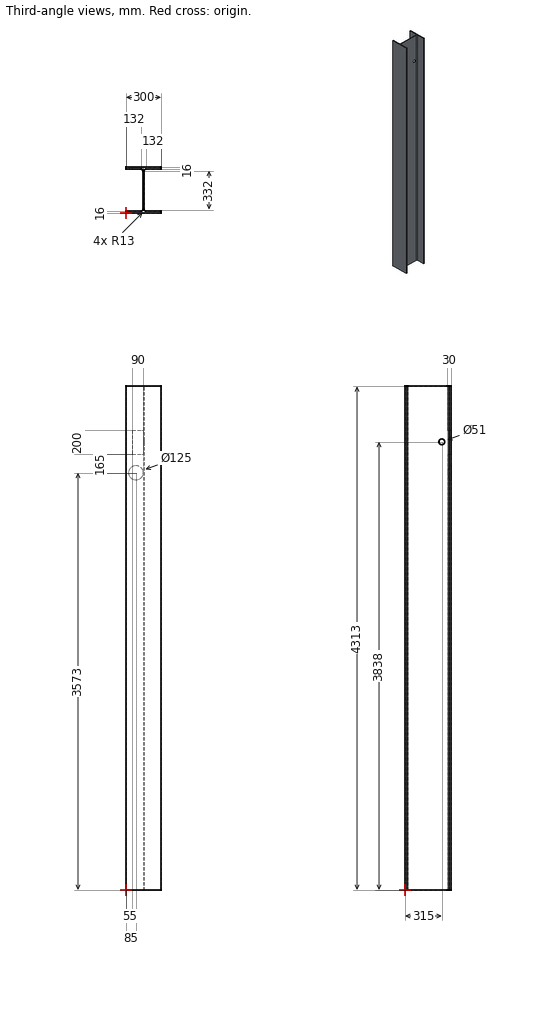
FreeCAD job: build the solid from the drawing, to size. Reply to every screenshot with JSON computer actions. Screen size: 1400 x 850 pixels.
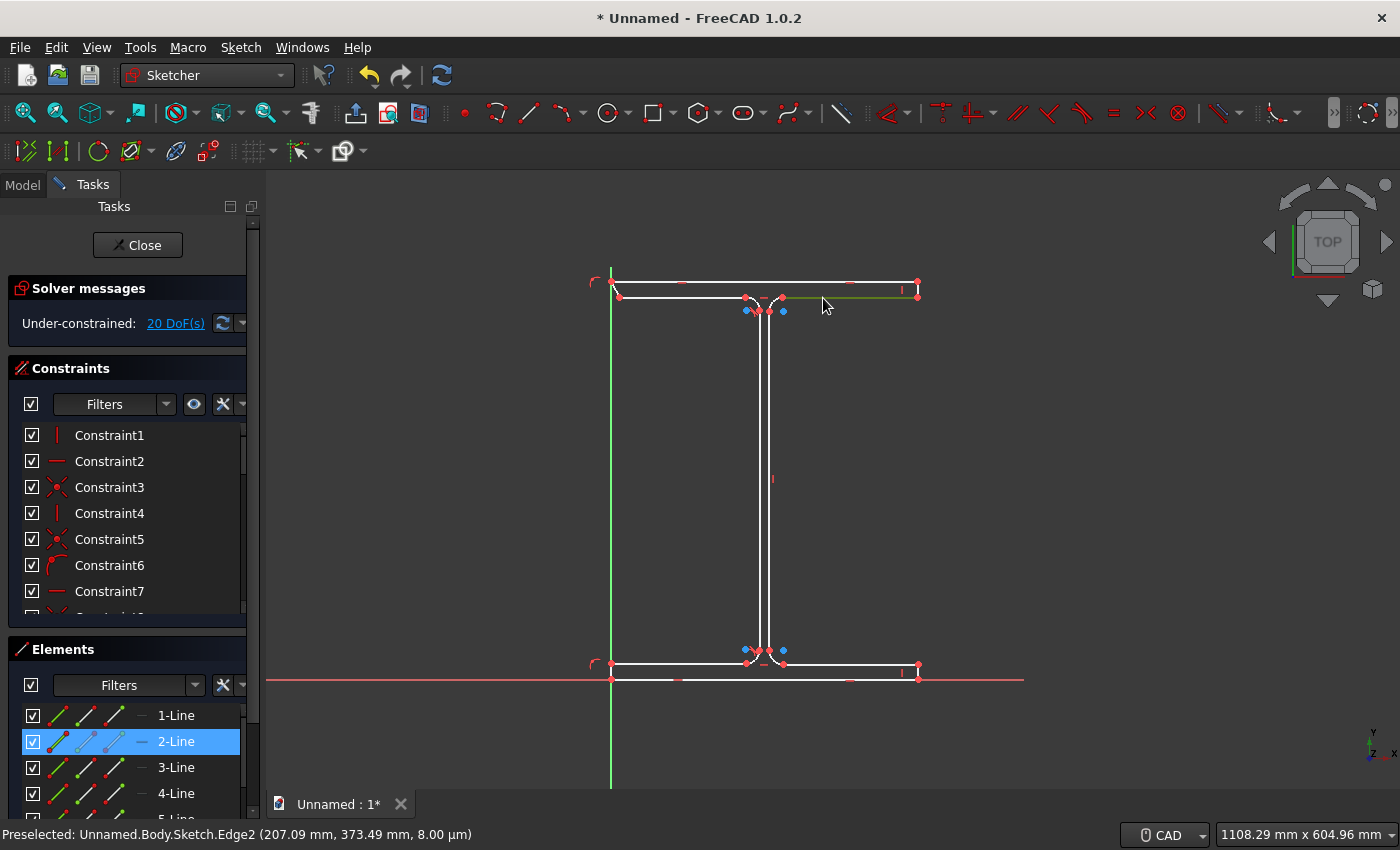
{"action": "scroll", "coordinate": [773, 302], "scroll_direction": "up", "scroll_amount": 2}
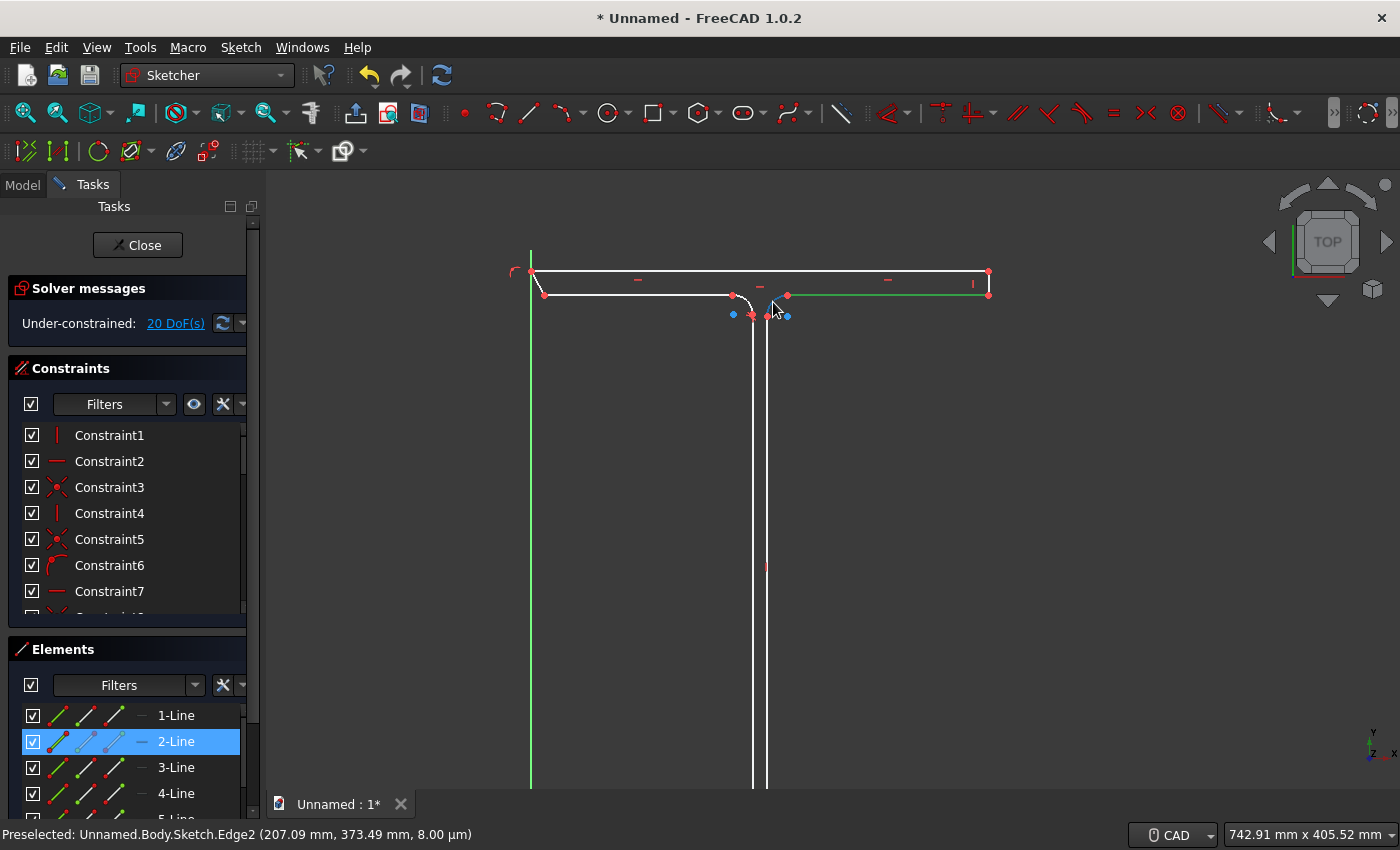
{"action": "left_click", "coordinate": [773, 302]}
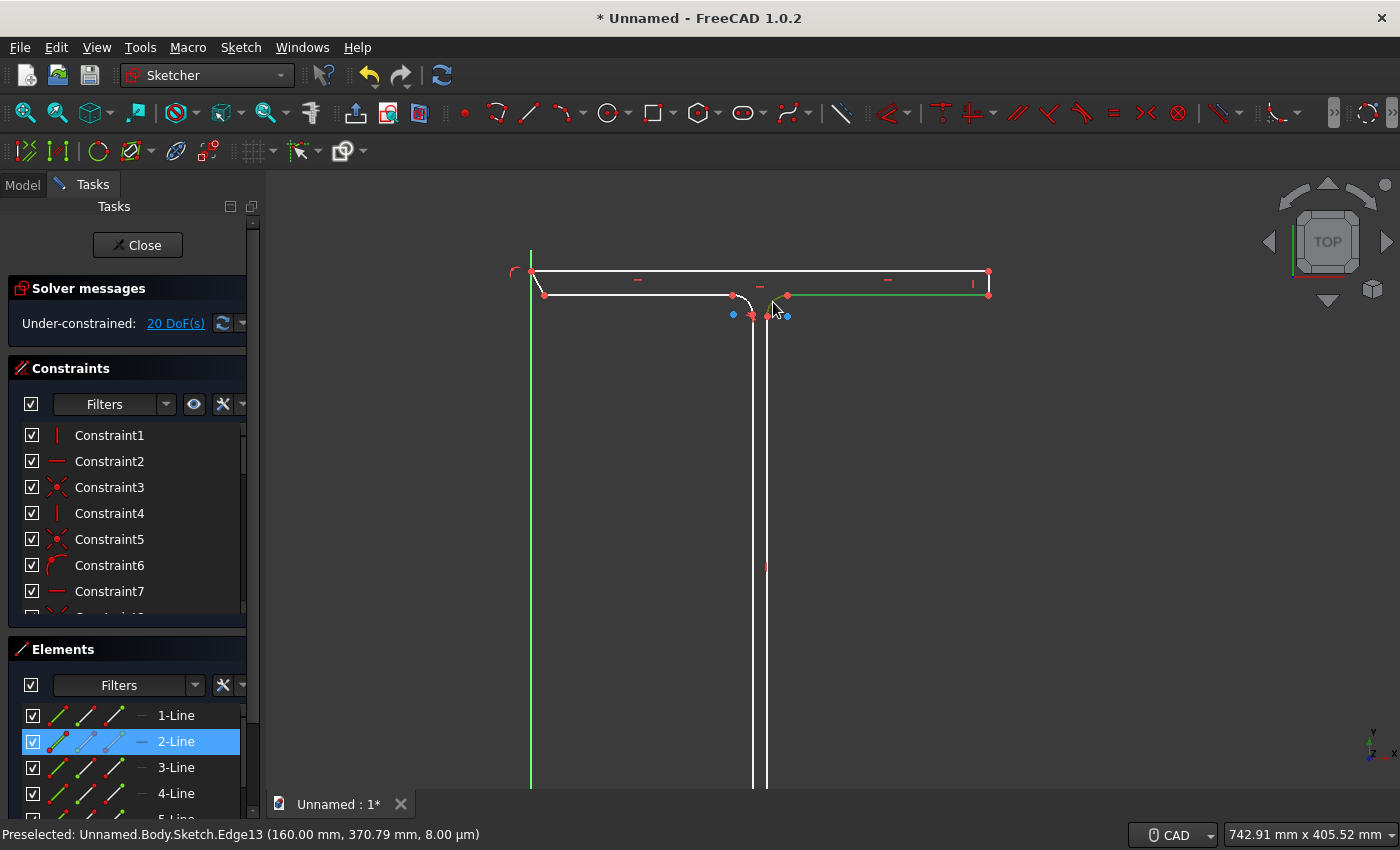
{"action": "left_click", "coordinate": [1082, 114]}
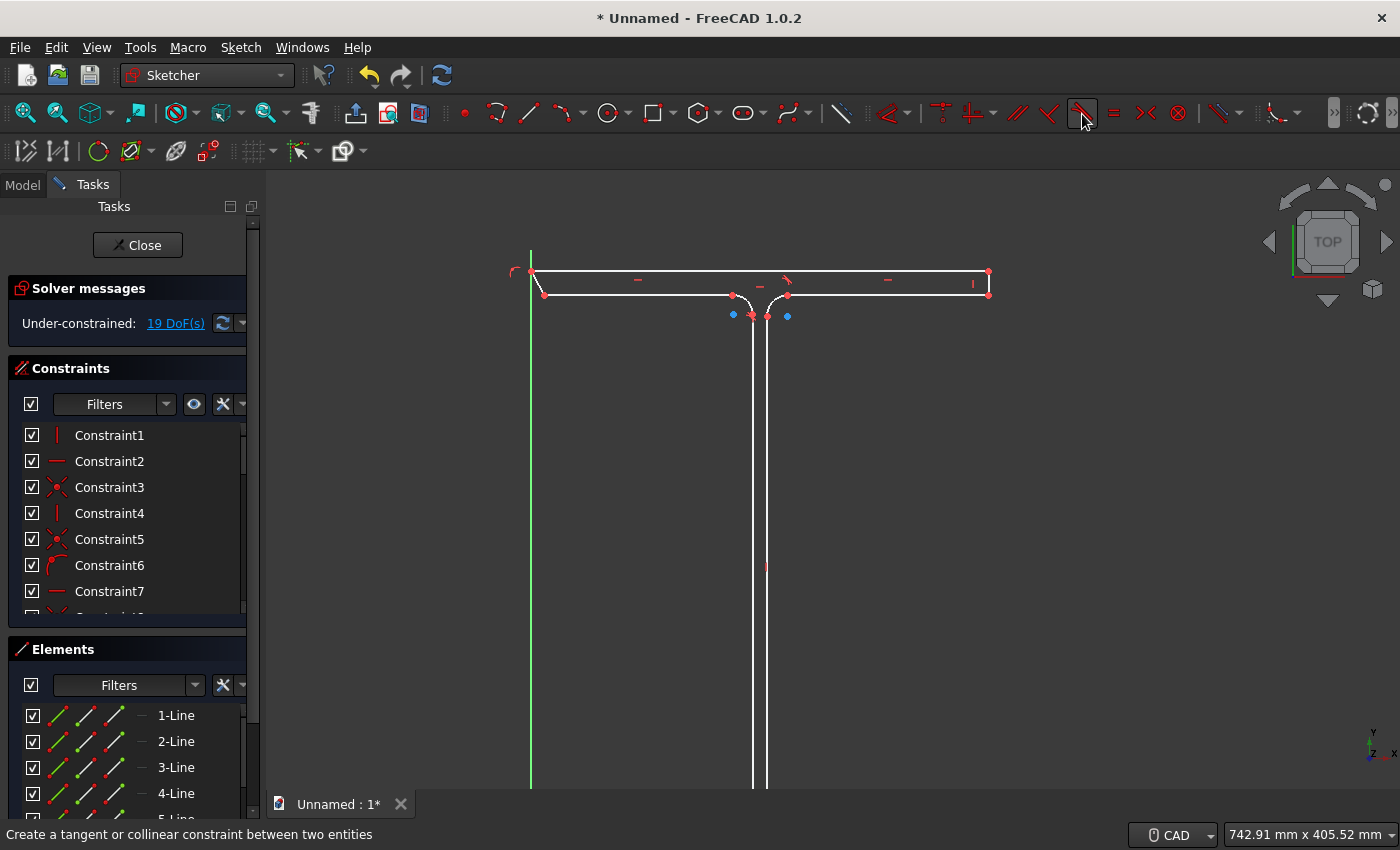
{"action": "left_click", "coordinate": [601, 295]}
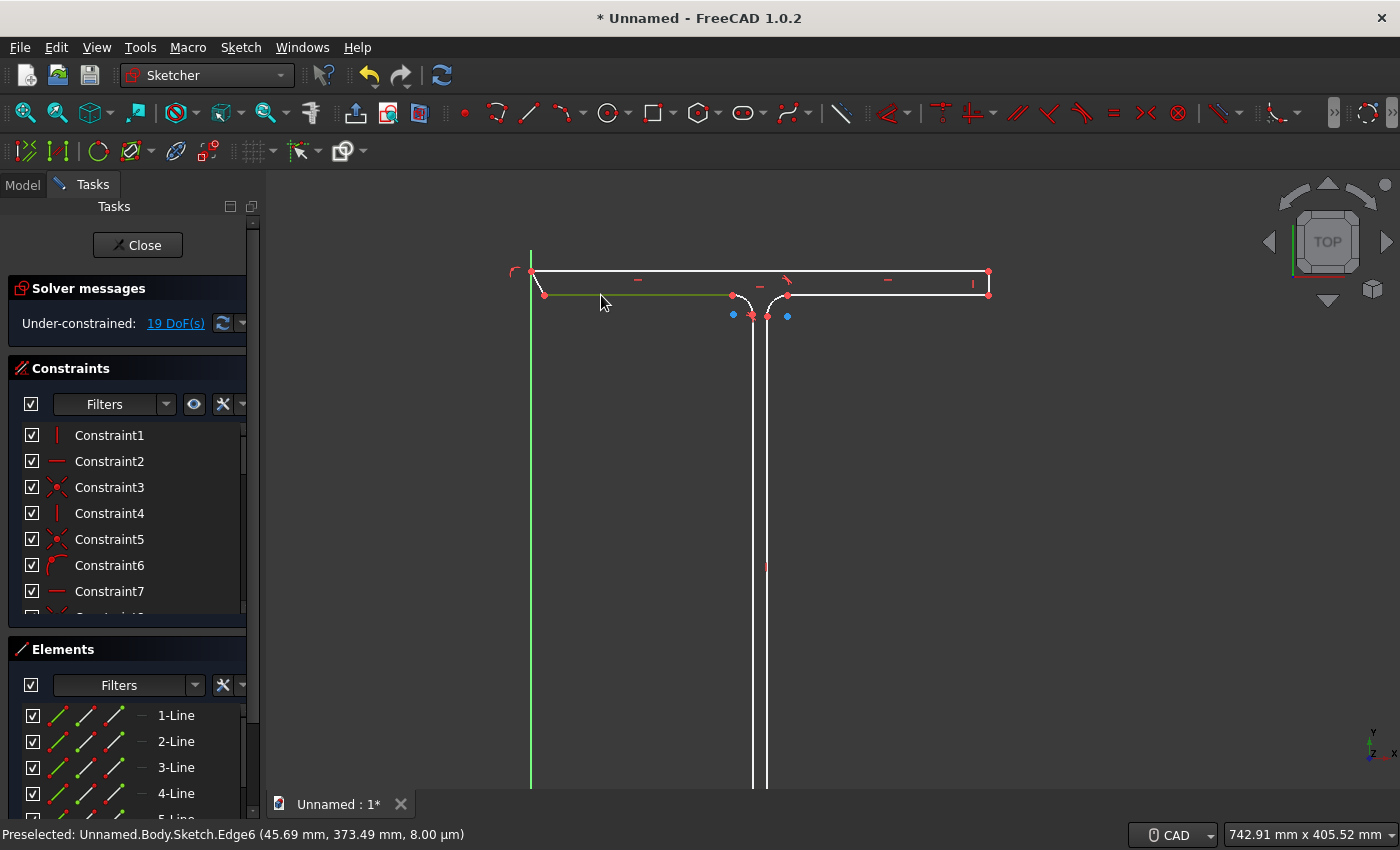
{"action": "scroll", "coordinate": [751, 306], "scroll_direction": "up", "scroll_amount": 2}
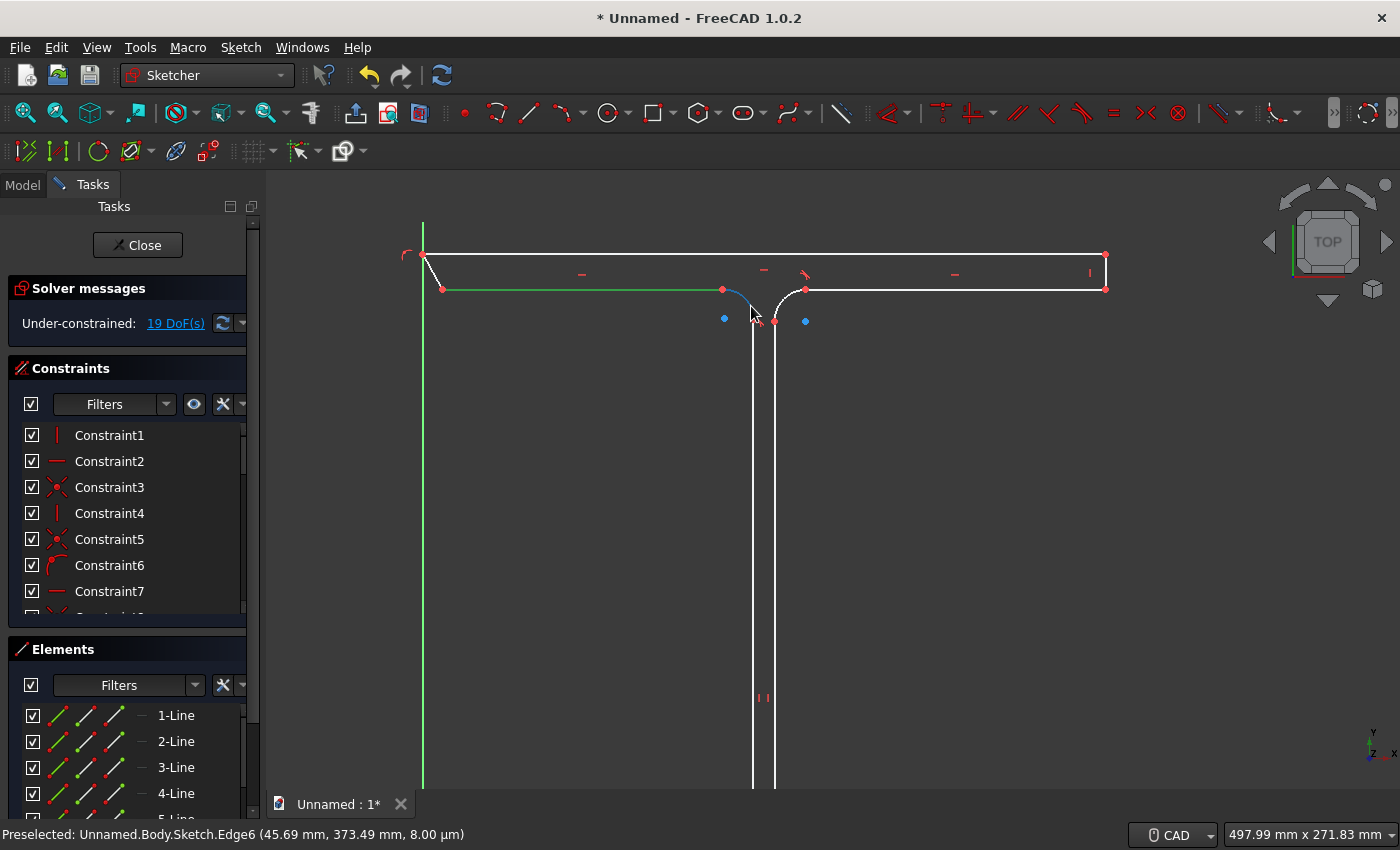
{"action": "left_click", "coordinate": [750, 305]}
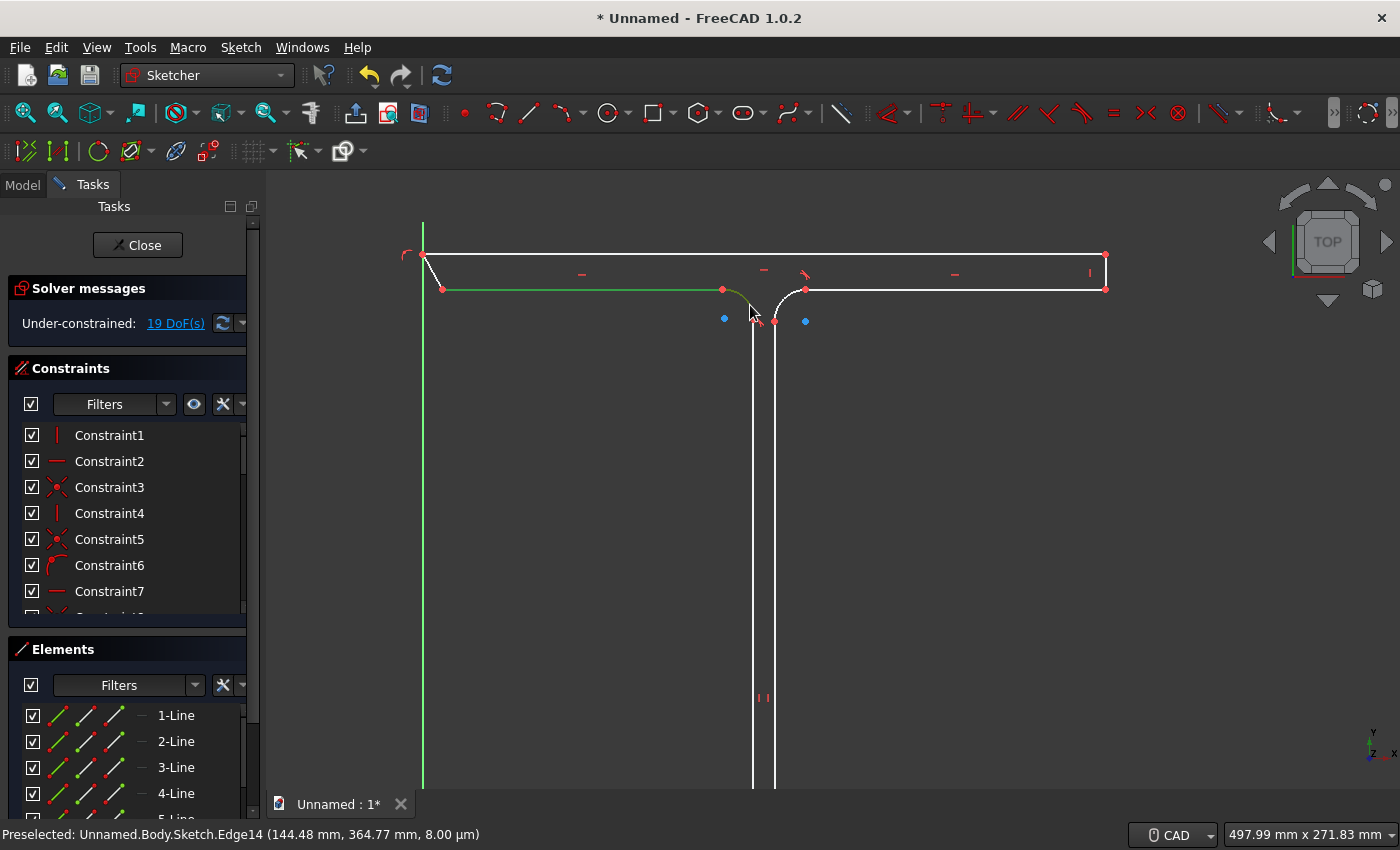
{"action": "left_click", "coordinate": [1082, 114]}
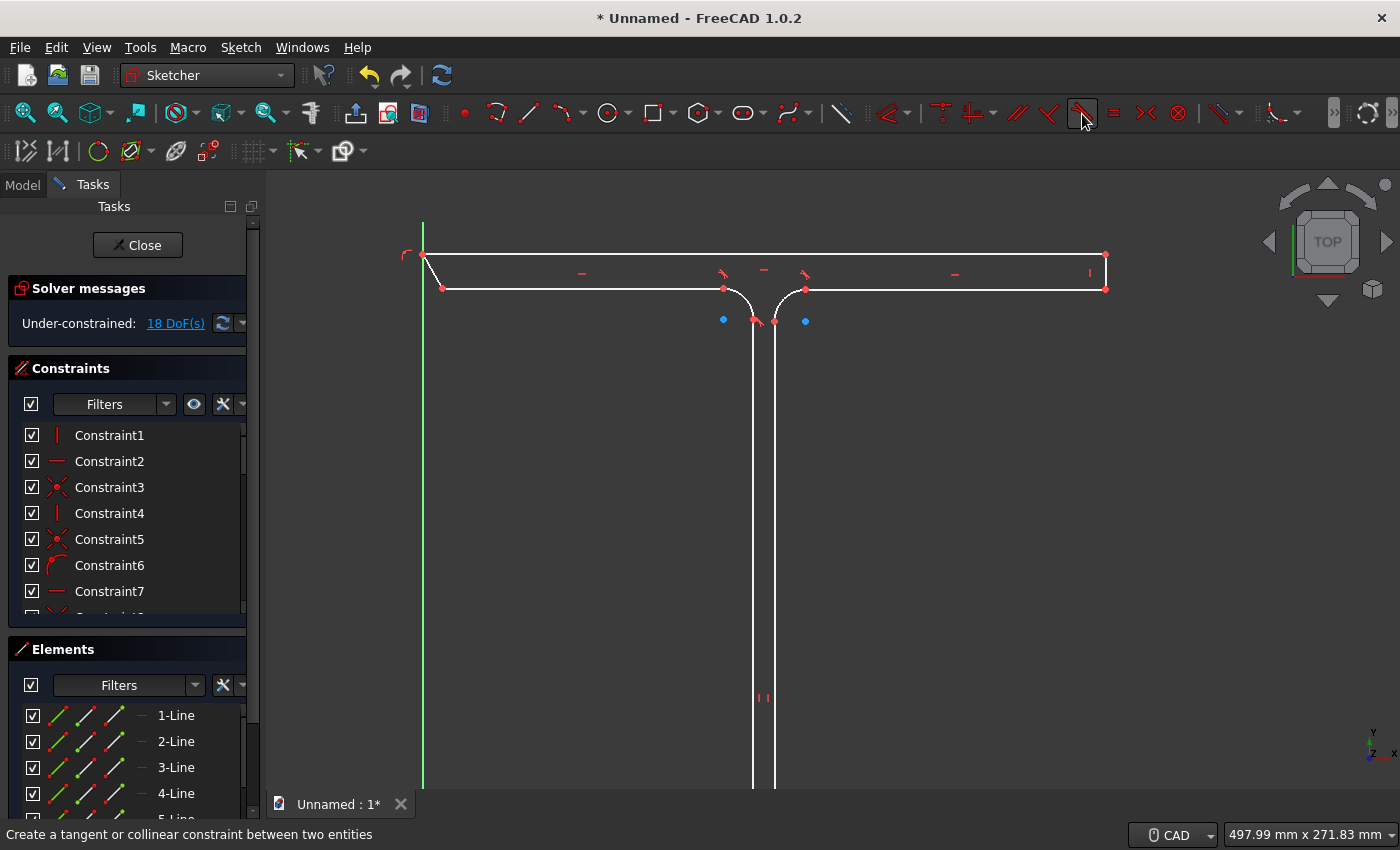
{"action": "left_click", "coordinate": [753, 546]}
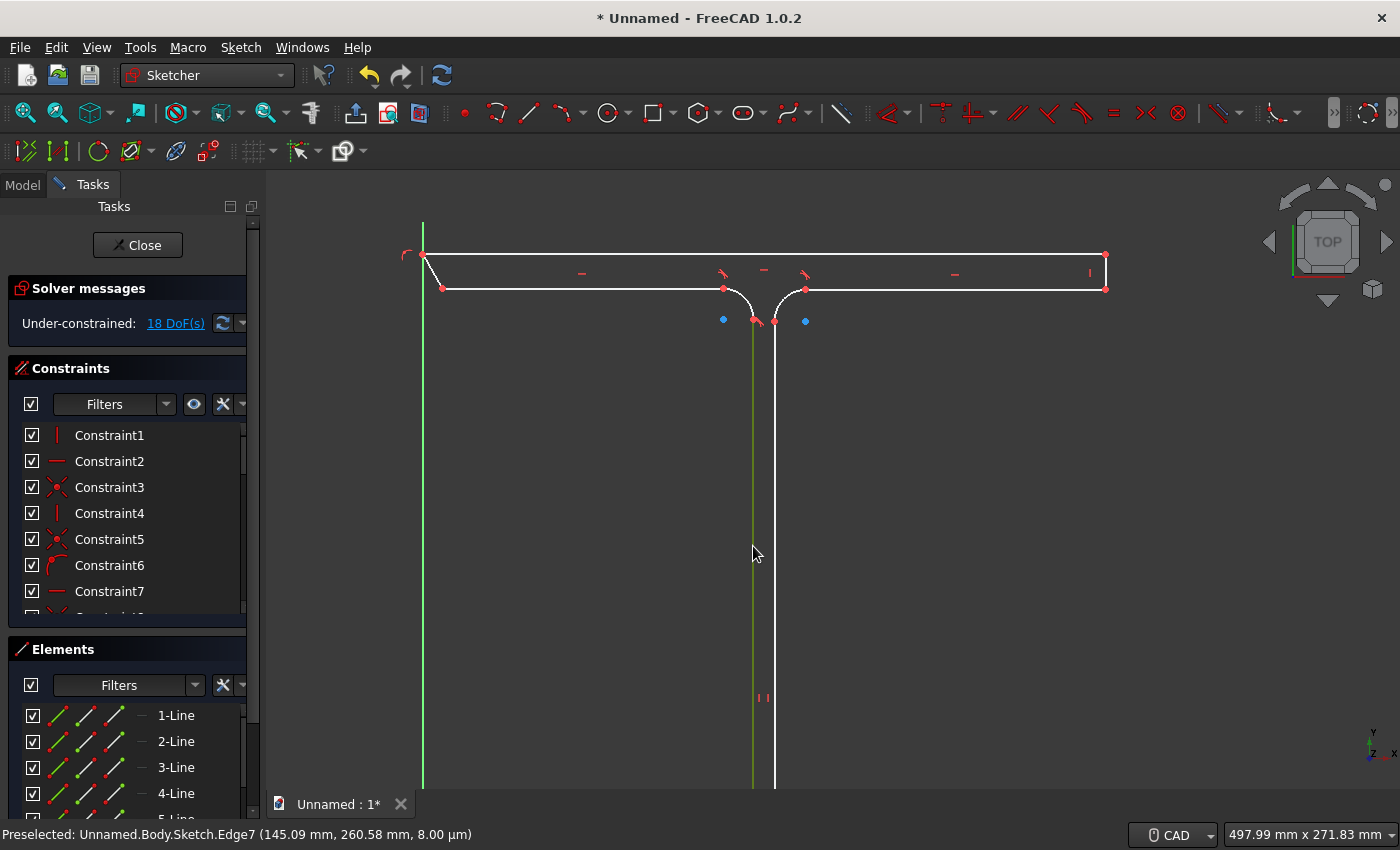
{"action": "left_click", "coordinate": [750, 305]}